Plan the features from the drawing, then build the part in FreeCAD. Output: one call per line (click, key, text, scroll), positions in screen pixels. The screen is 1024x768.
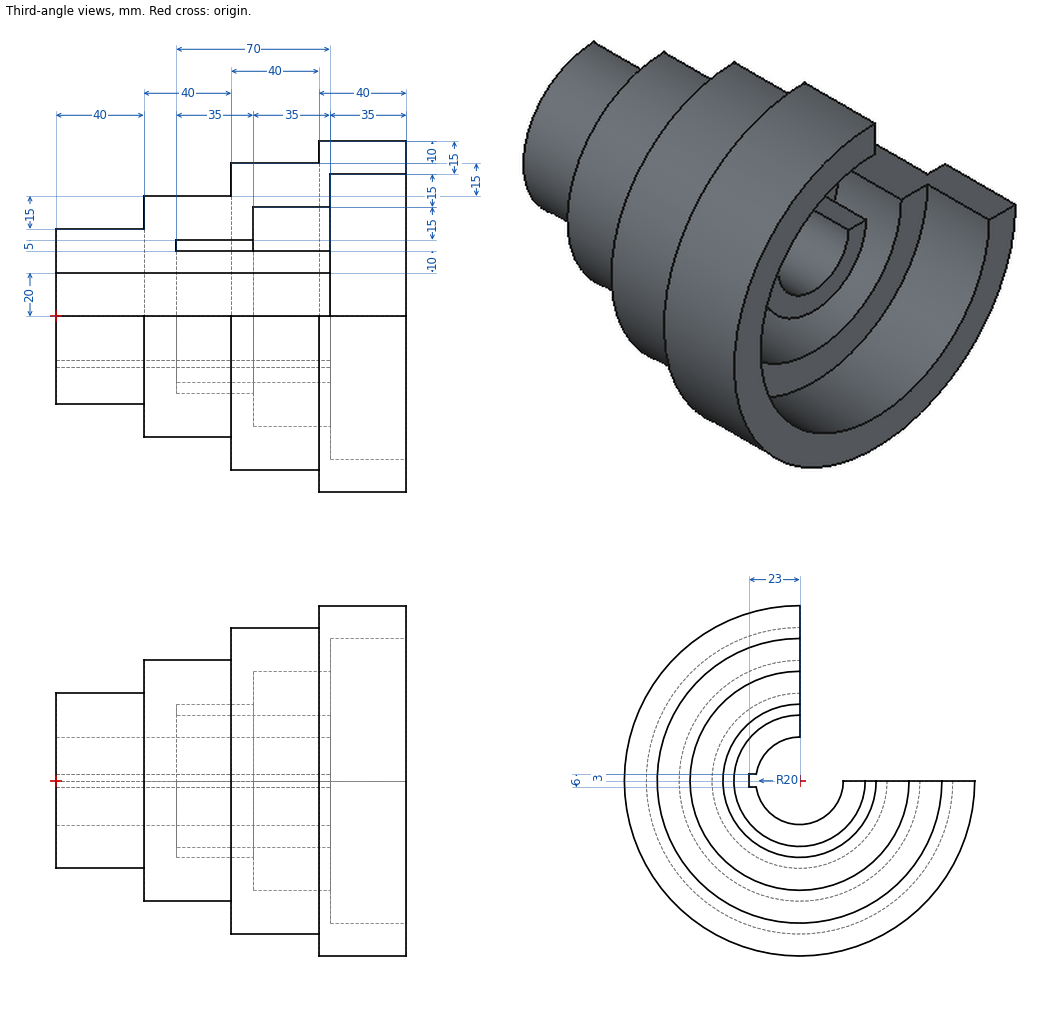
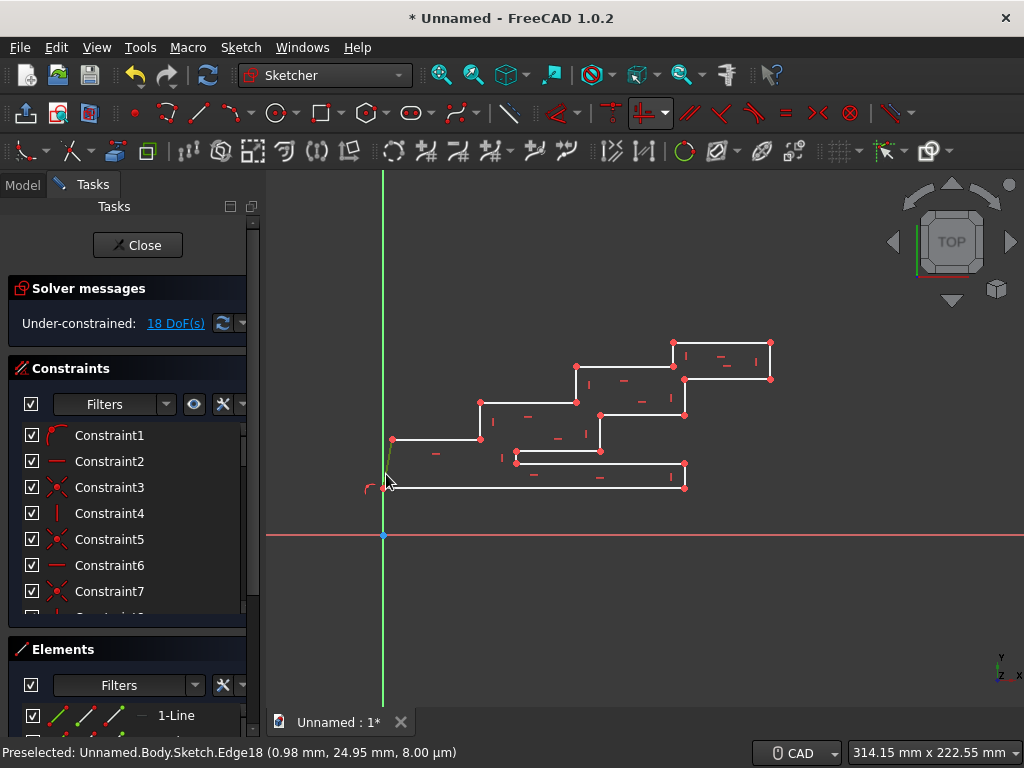
key(v)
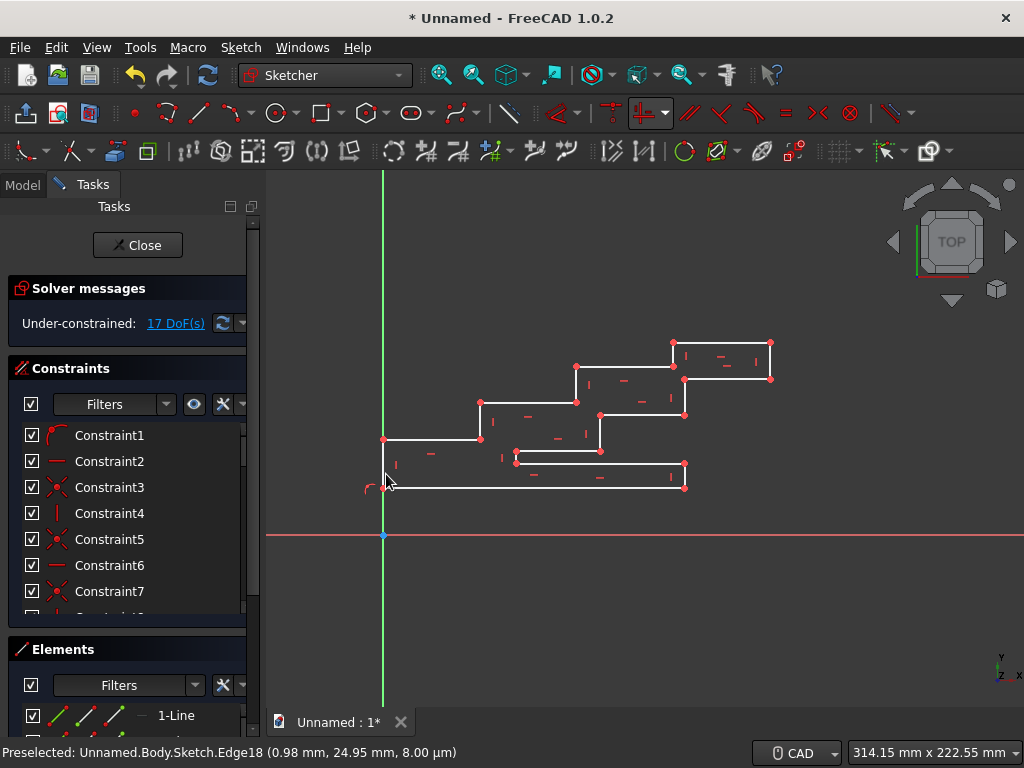
scroll(516, 458, up, 6)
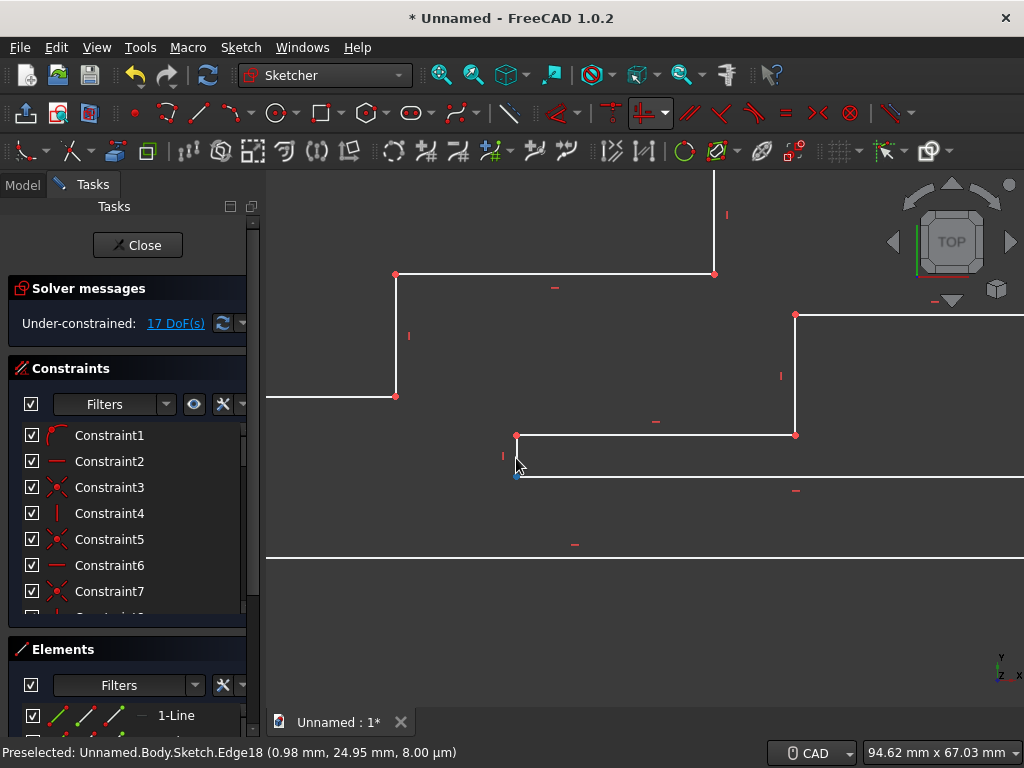
click(517, 456)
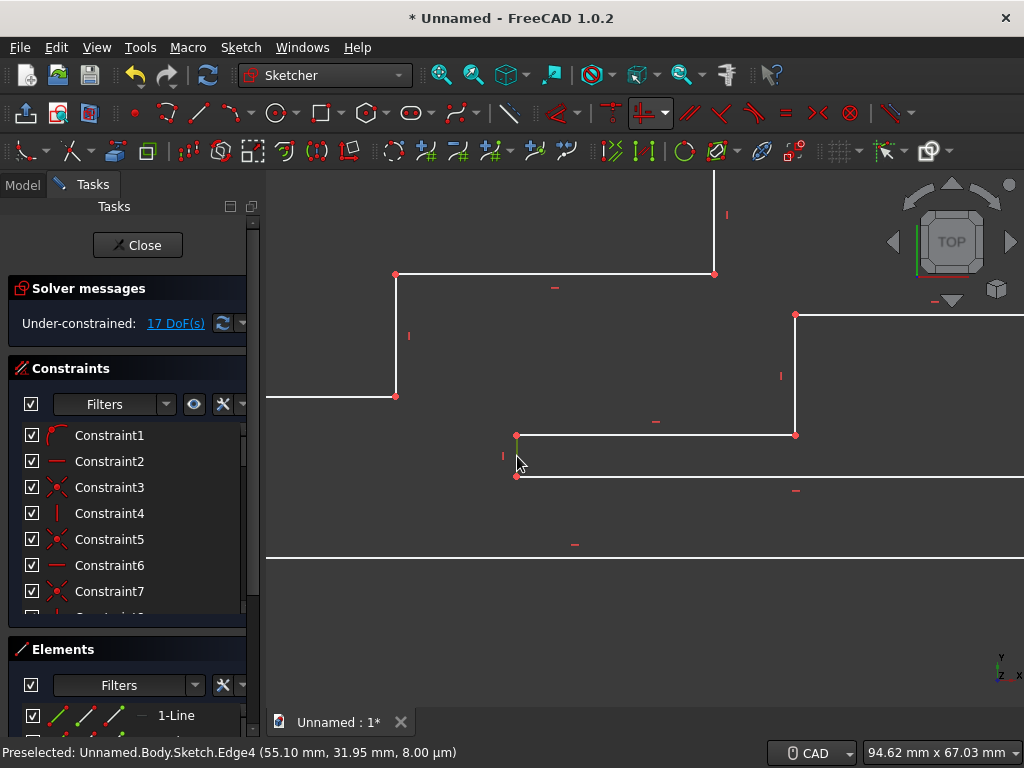
key(i)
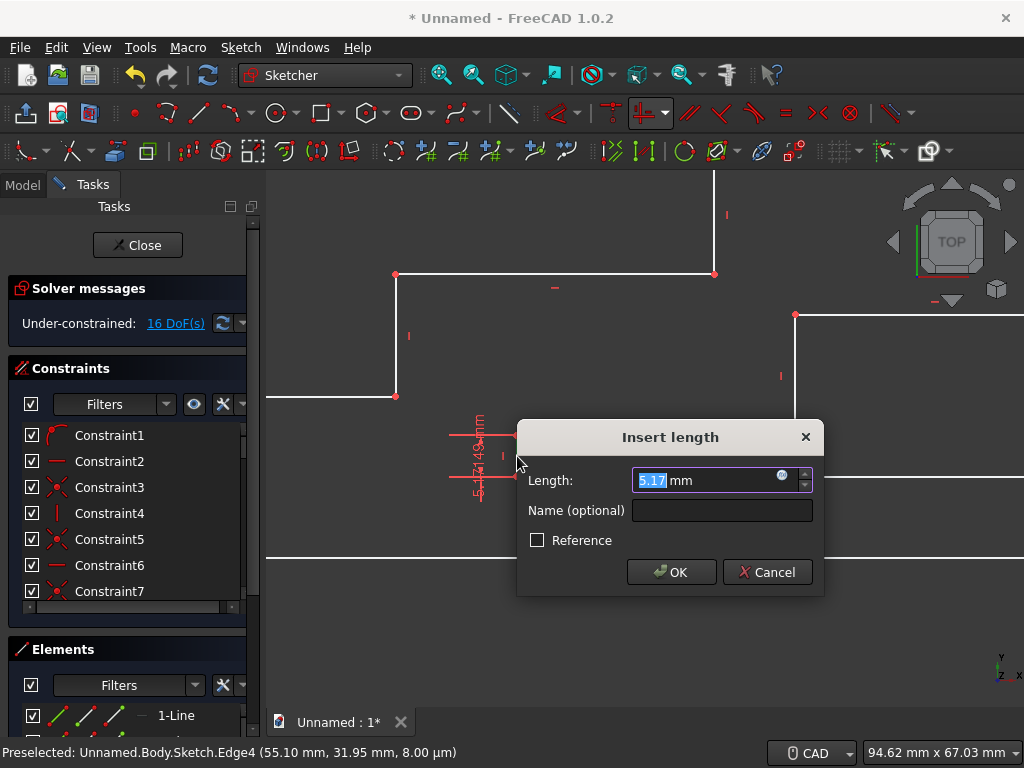
text(5)
key(Return)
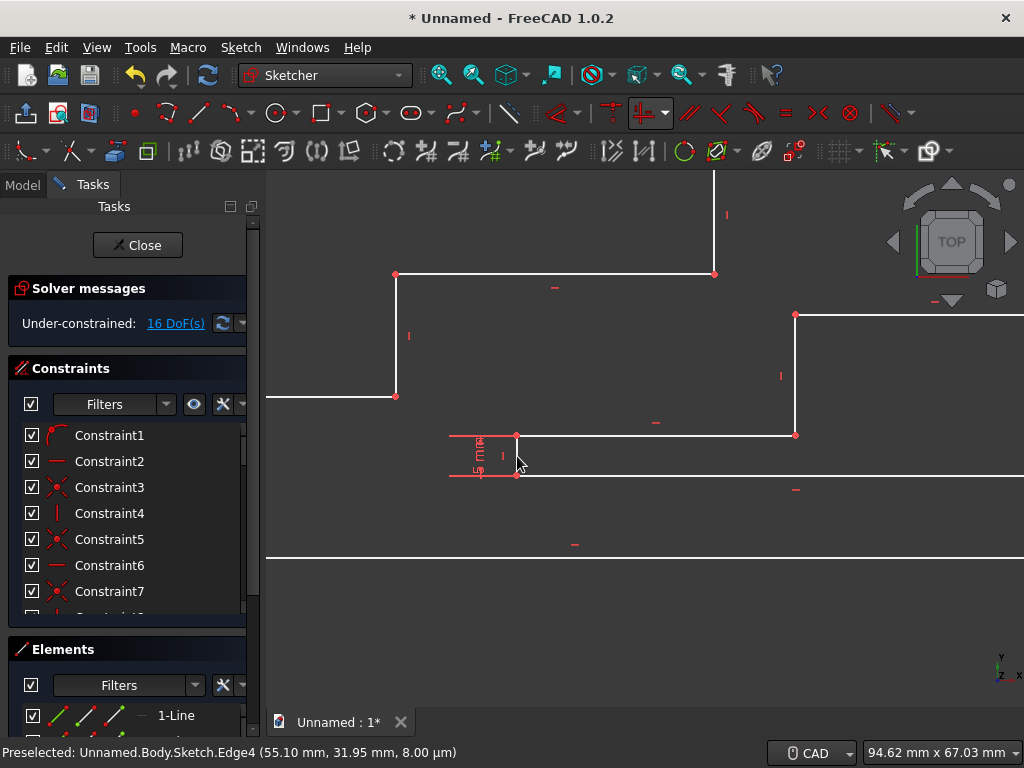
scroll(516, 458, down, 6)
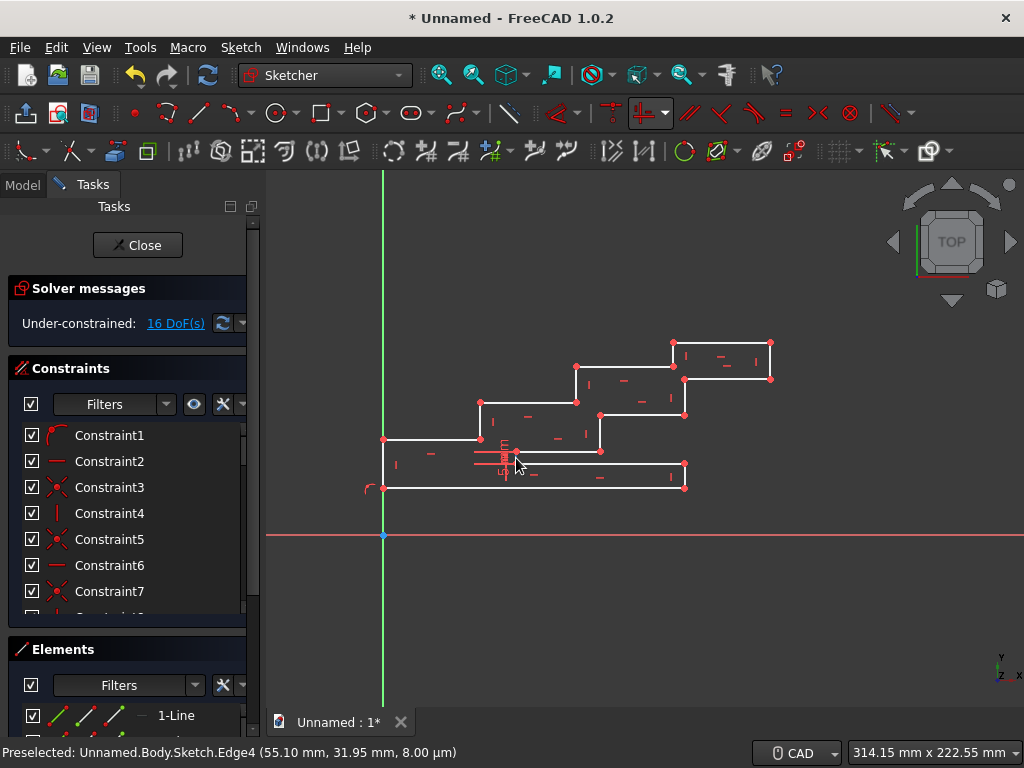
scroll(685, 481, up, 4)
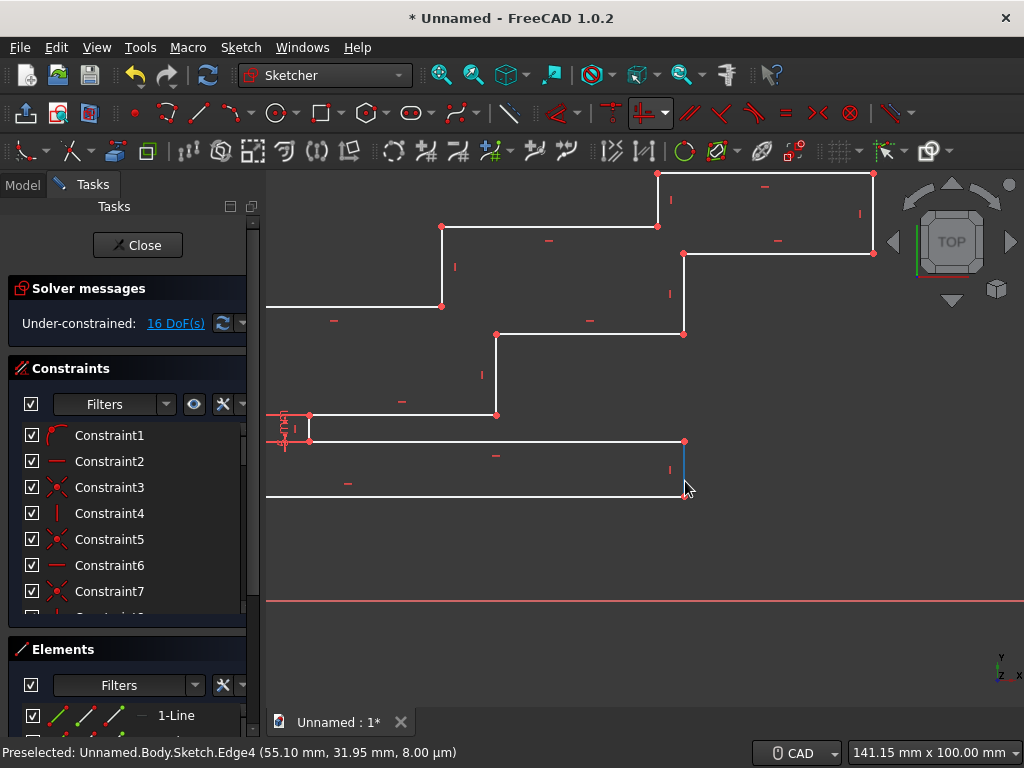
click(684, 480)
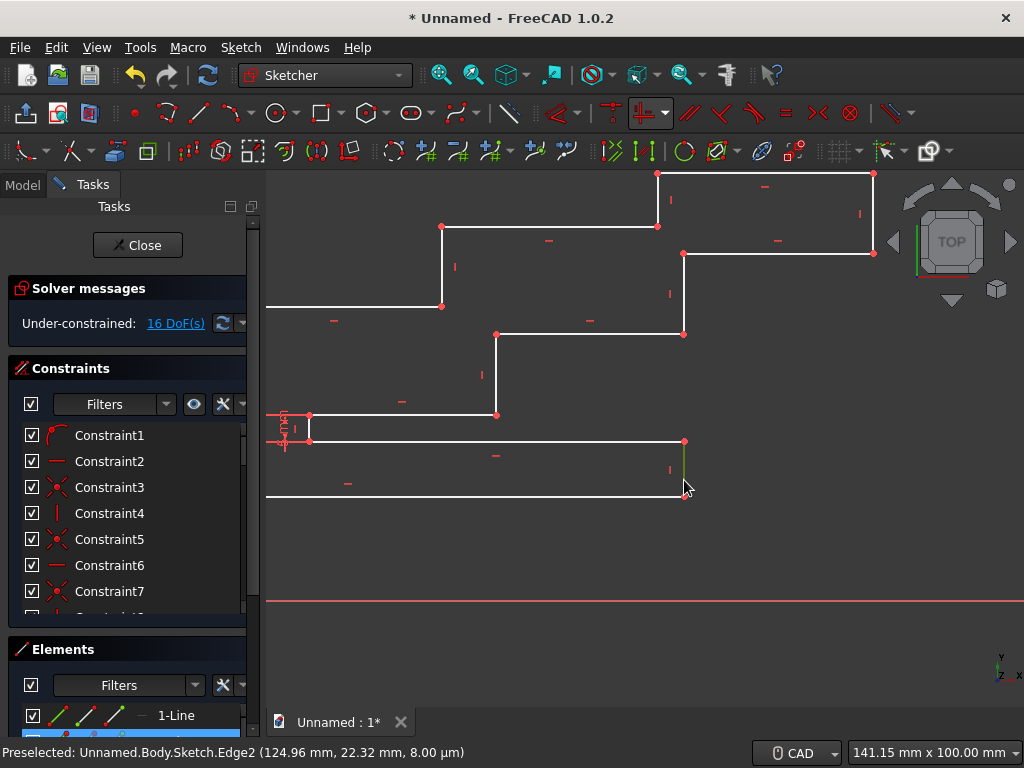
key(i)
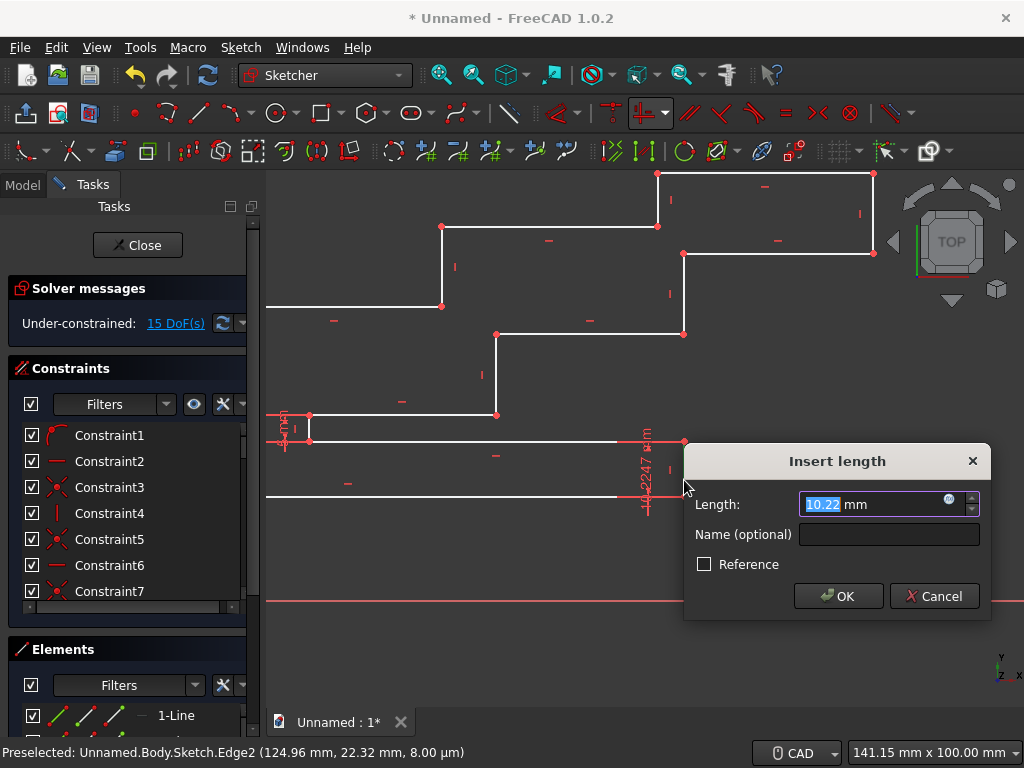
text(10)
key(Return)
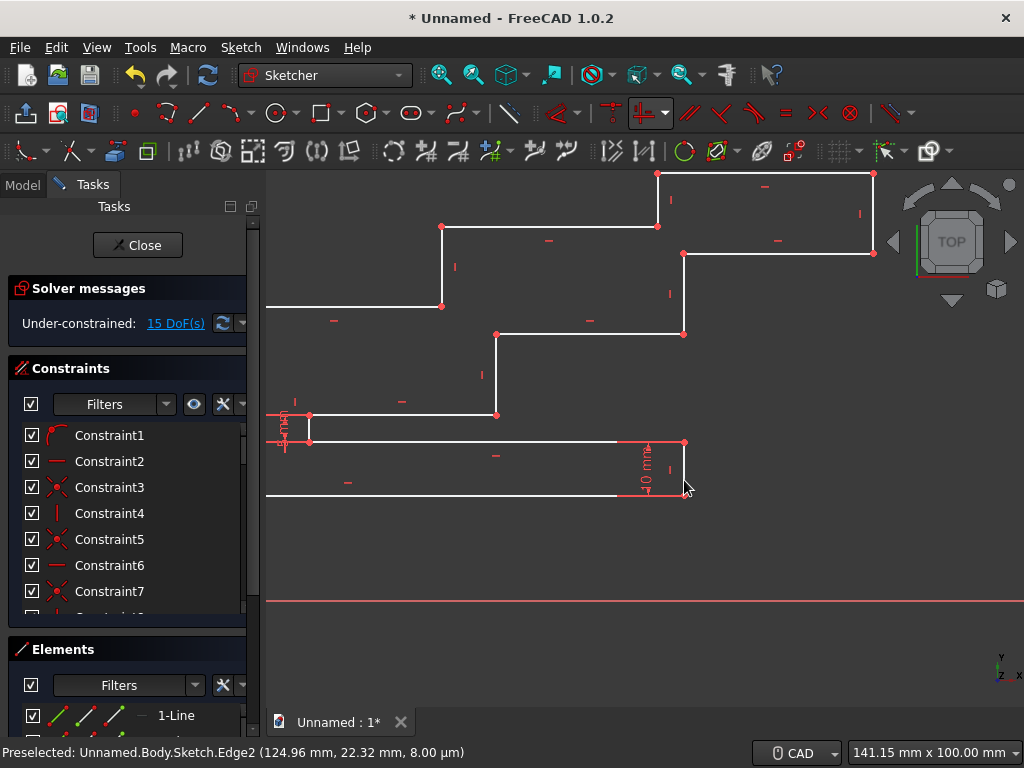
click(572, 442)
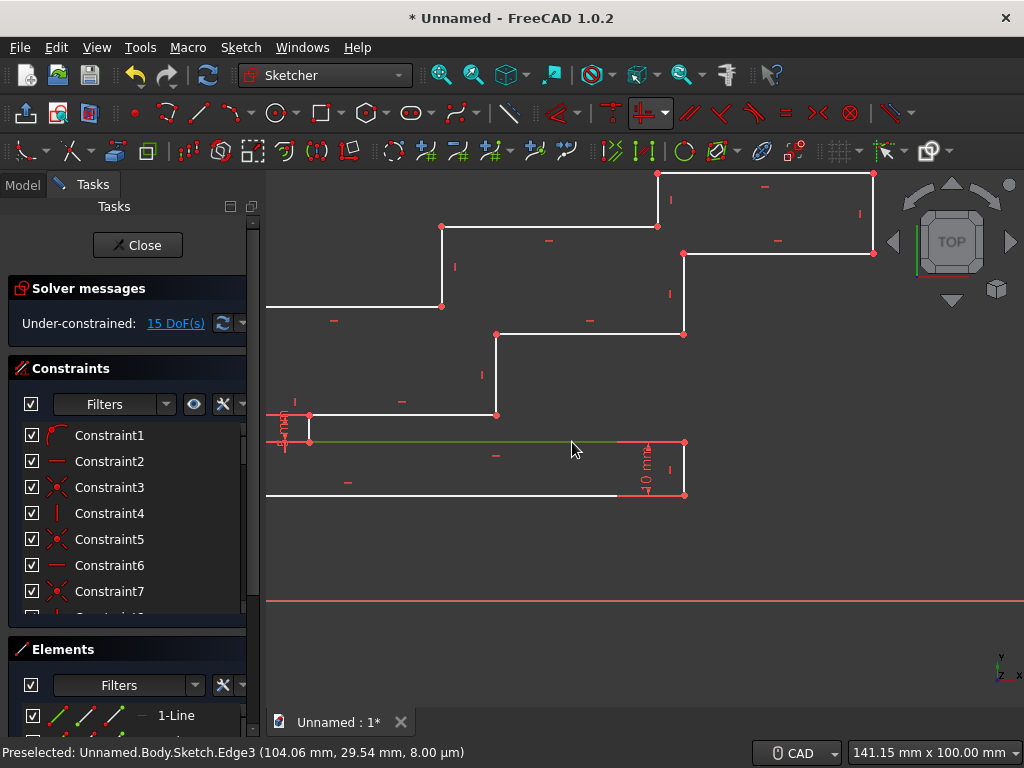
key(l)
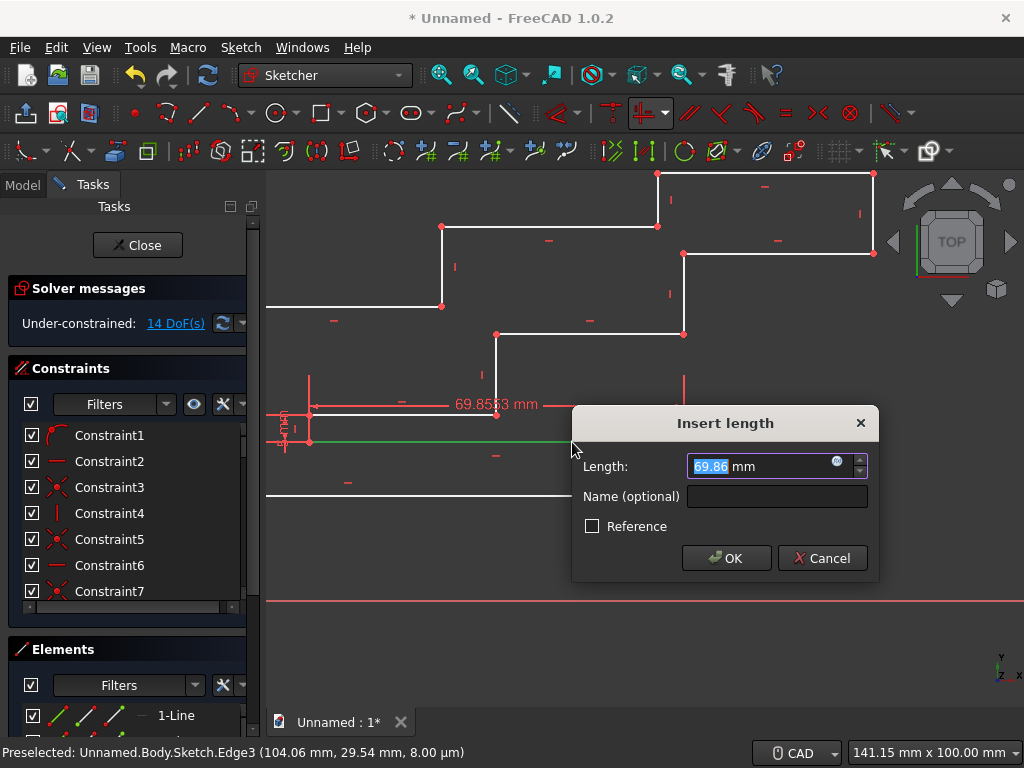
text(70)
key(Return)